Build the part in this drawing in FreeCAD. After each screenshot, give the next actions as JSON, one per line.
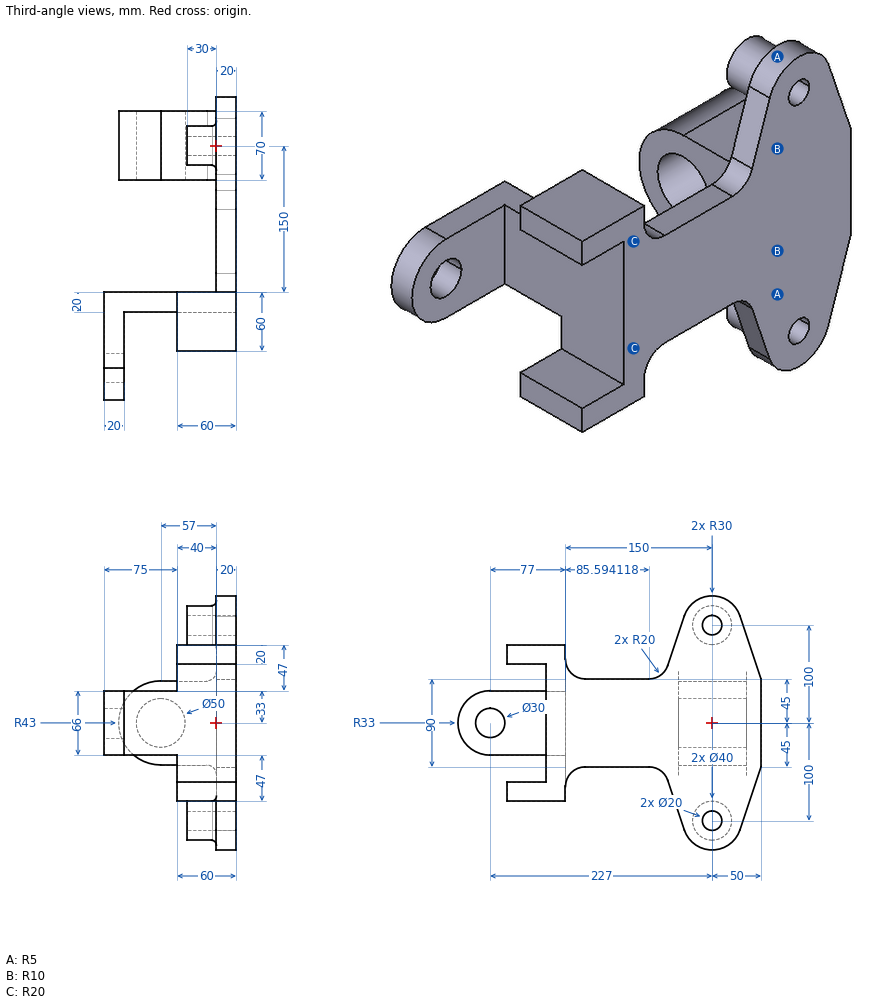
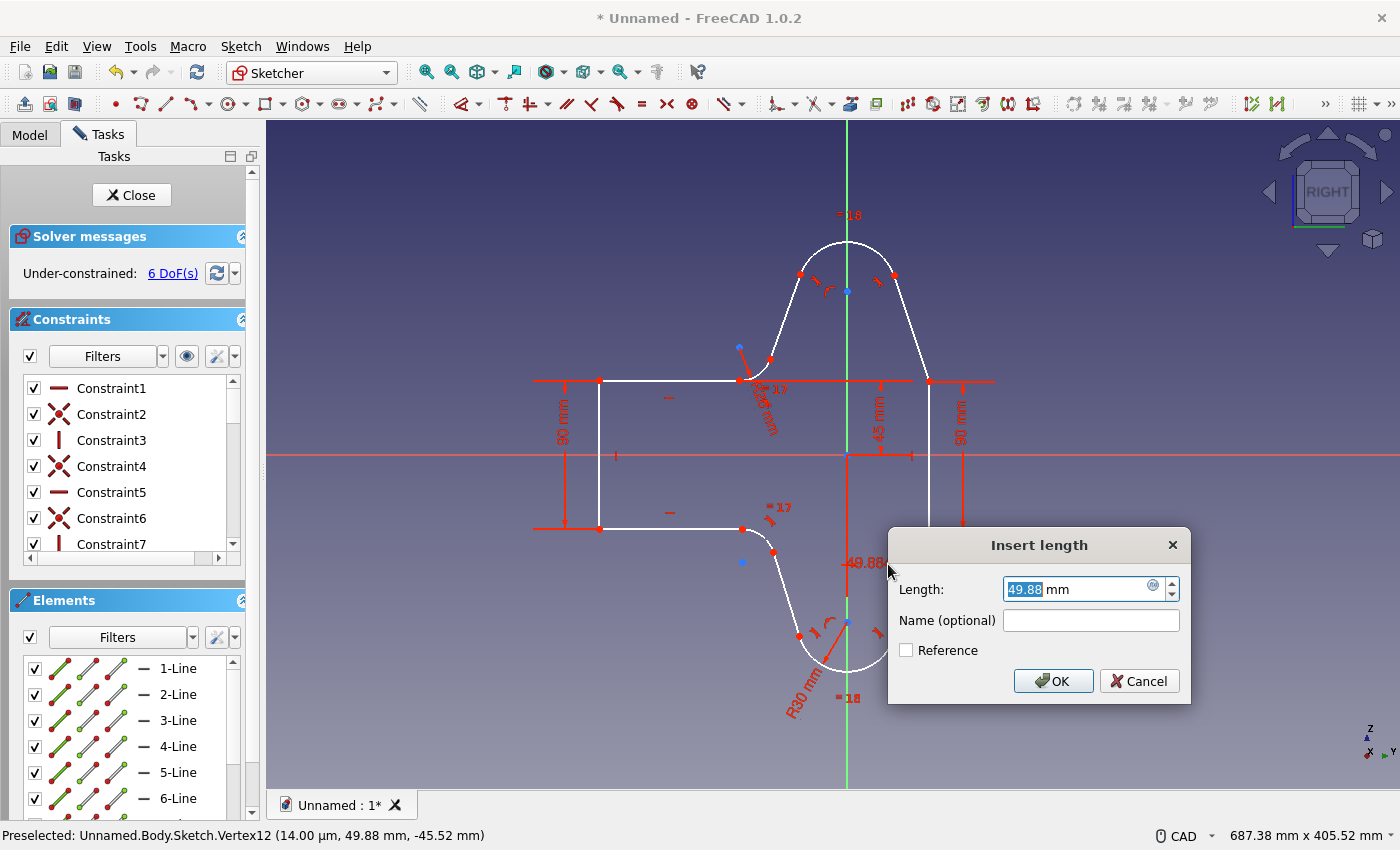
{"action": "type", "text": "50"}
{"action": "key", "text": "Return"}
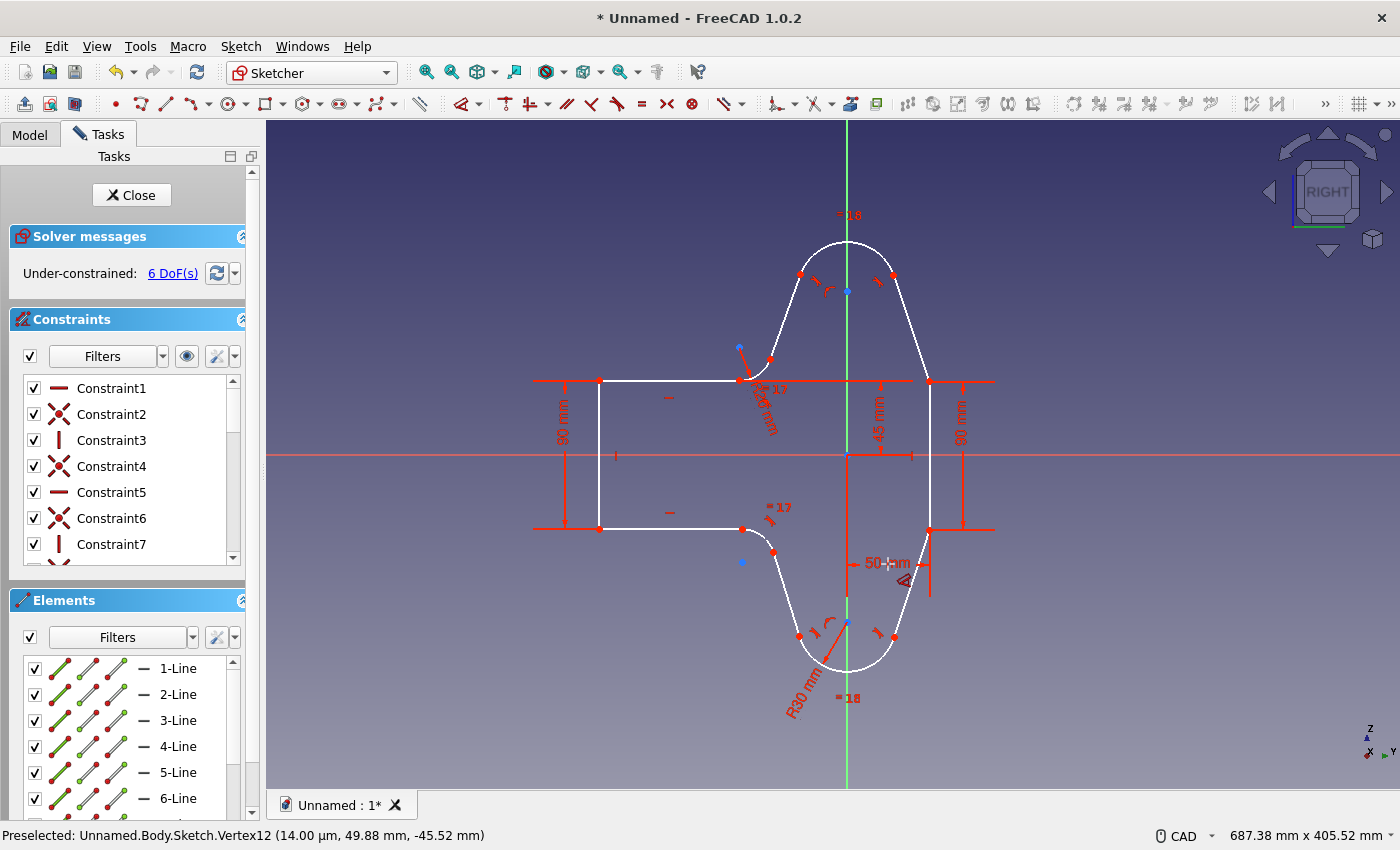
{"action": "left_click", "coordinate": [930, 530]}
{"action": "left_click", "coordinate": [964, 493]}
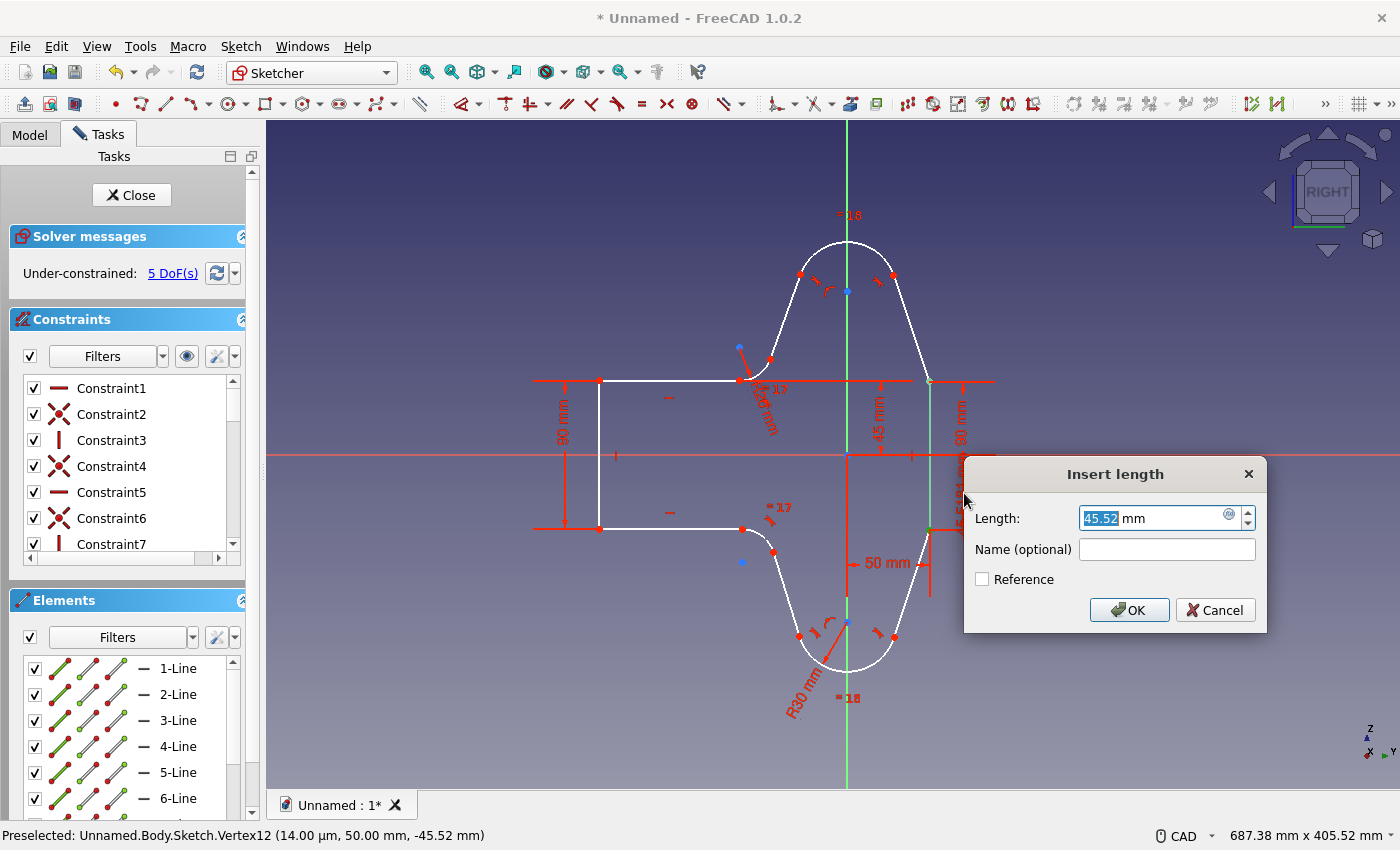
{"action": "type", "text": "45"}
{"action": "key", "text": "Return"}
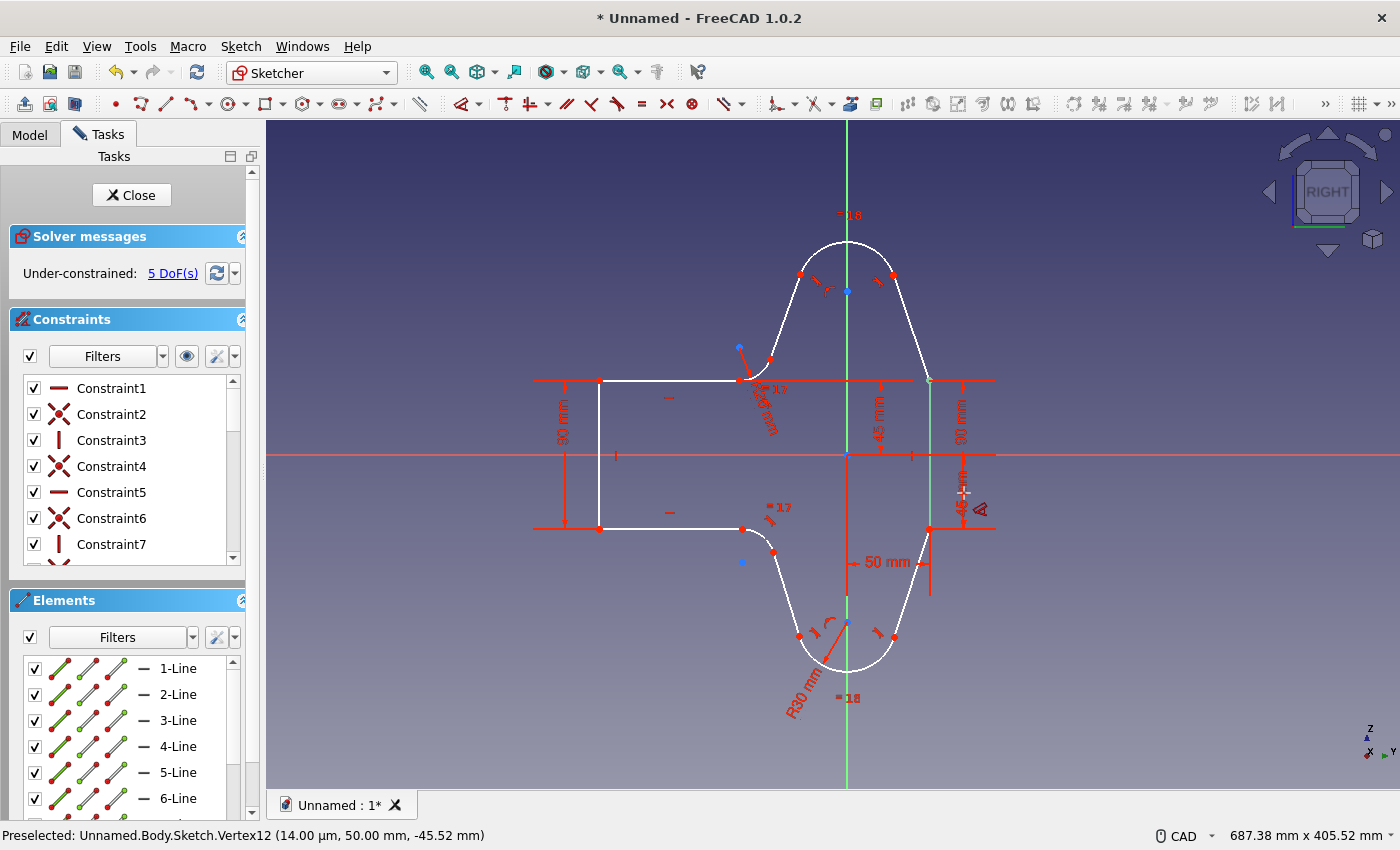
{"action": "left_click", "coordinate": [599, 381]}
{"action": "left_click", "coordinate": [723, 347]}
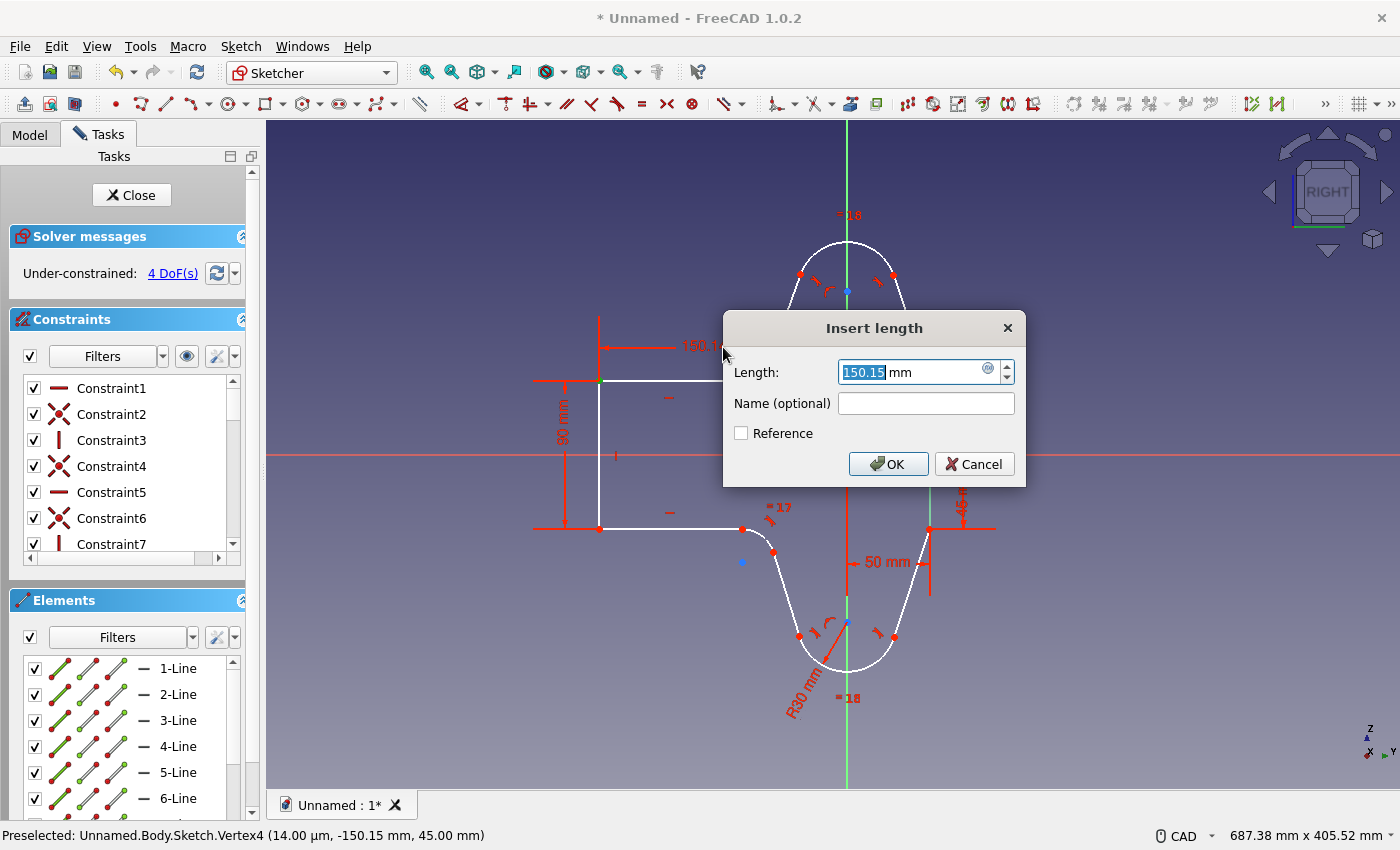
{"action": "type", "text": "150"}
{"action": "key", "text": "Return"}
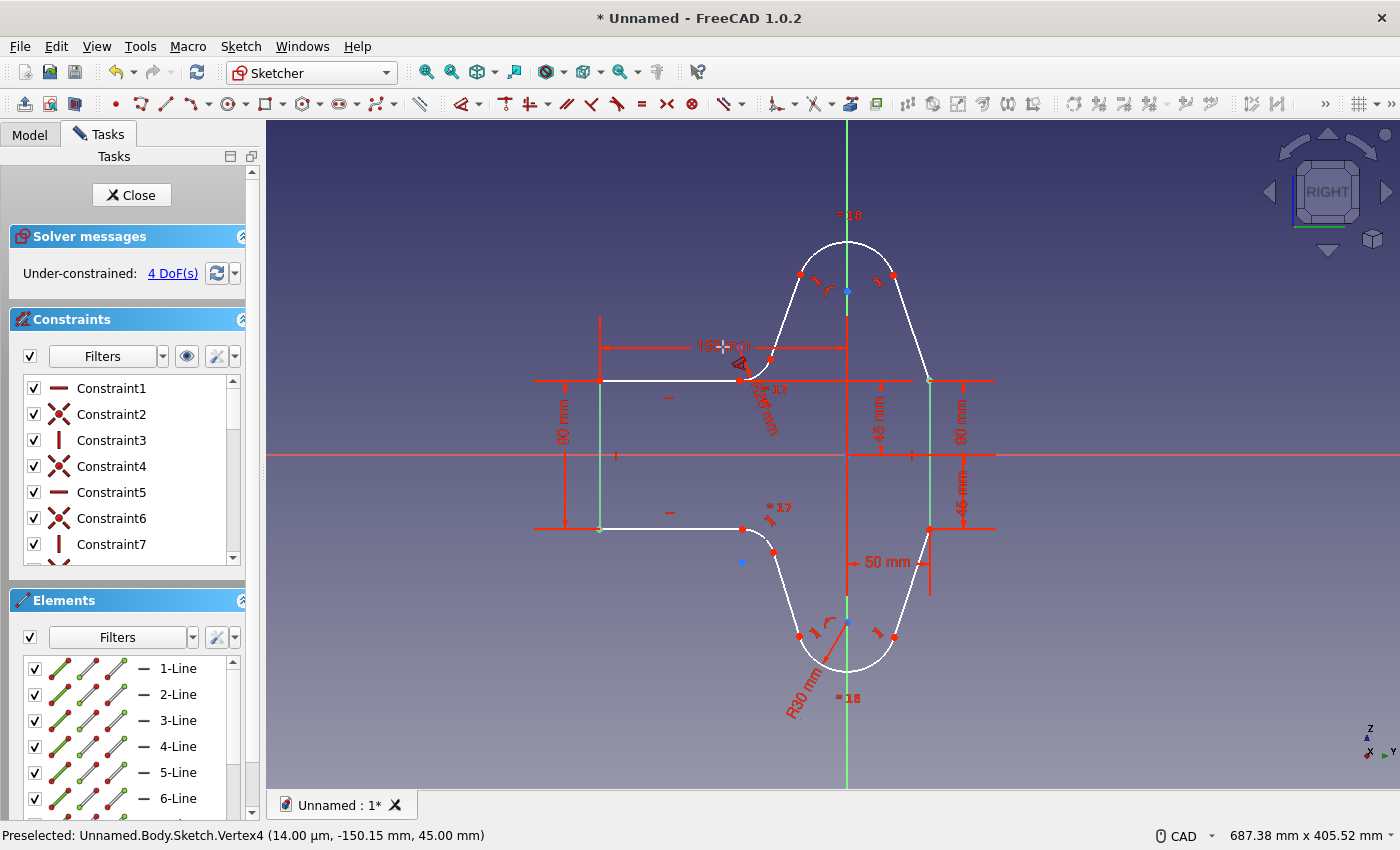
{"action": "left_click", "coordinate": [847, 622]}
{"action": "left_click", "coordinate": [881, 539]}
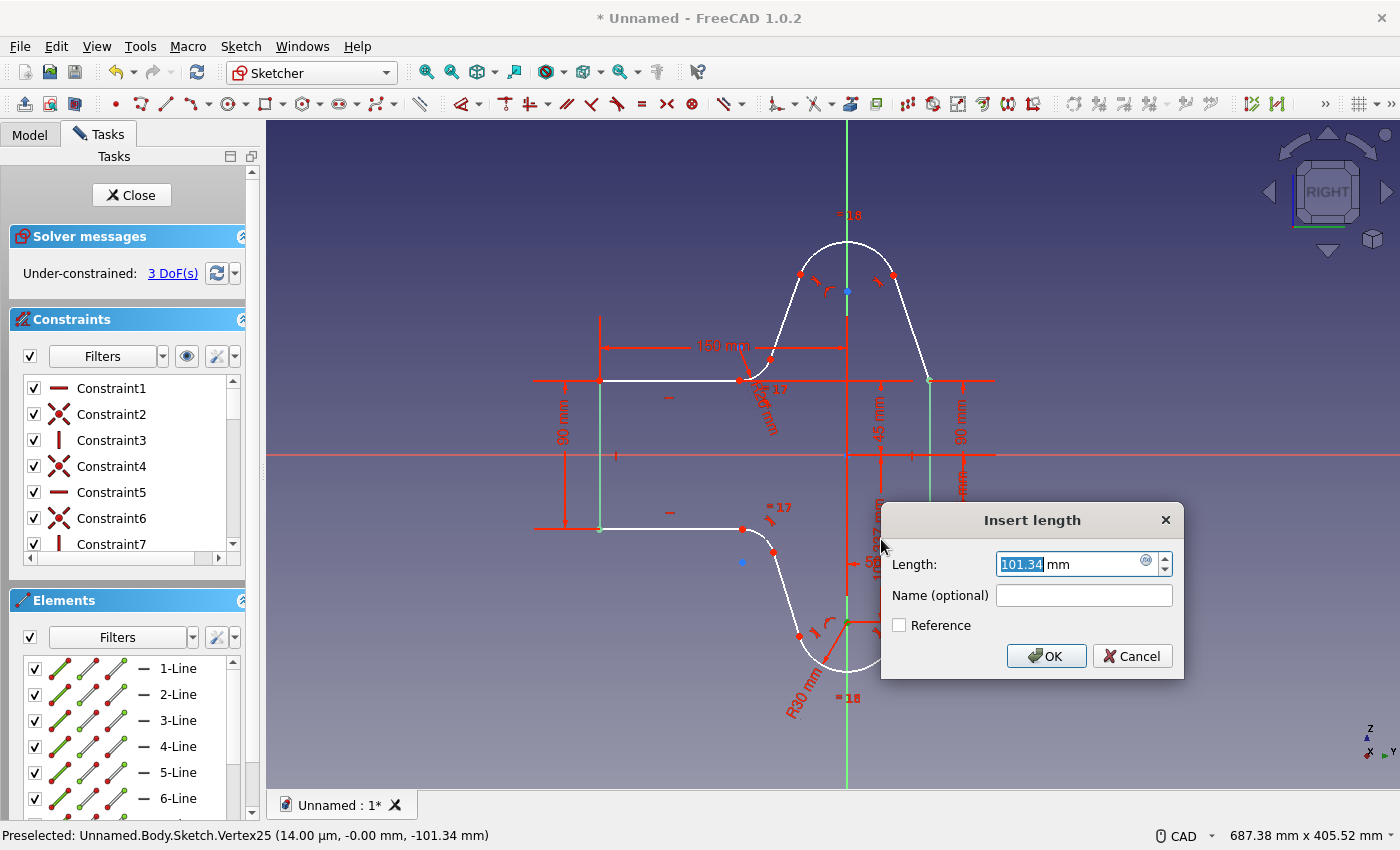
{"action": "type", "text": "100"}
{"action": "key", "text": "Return"}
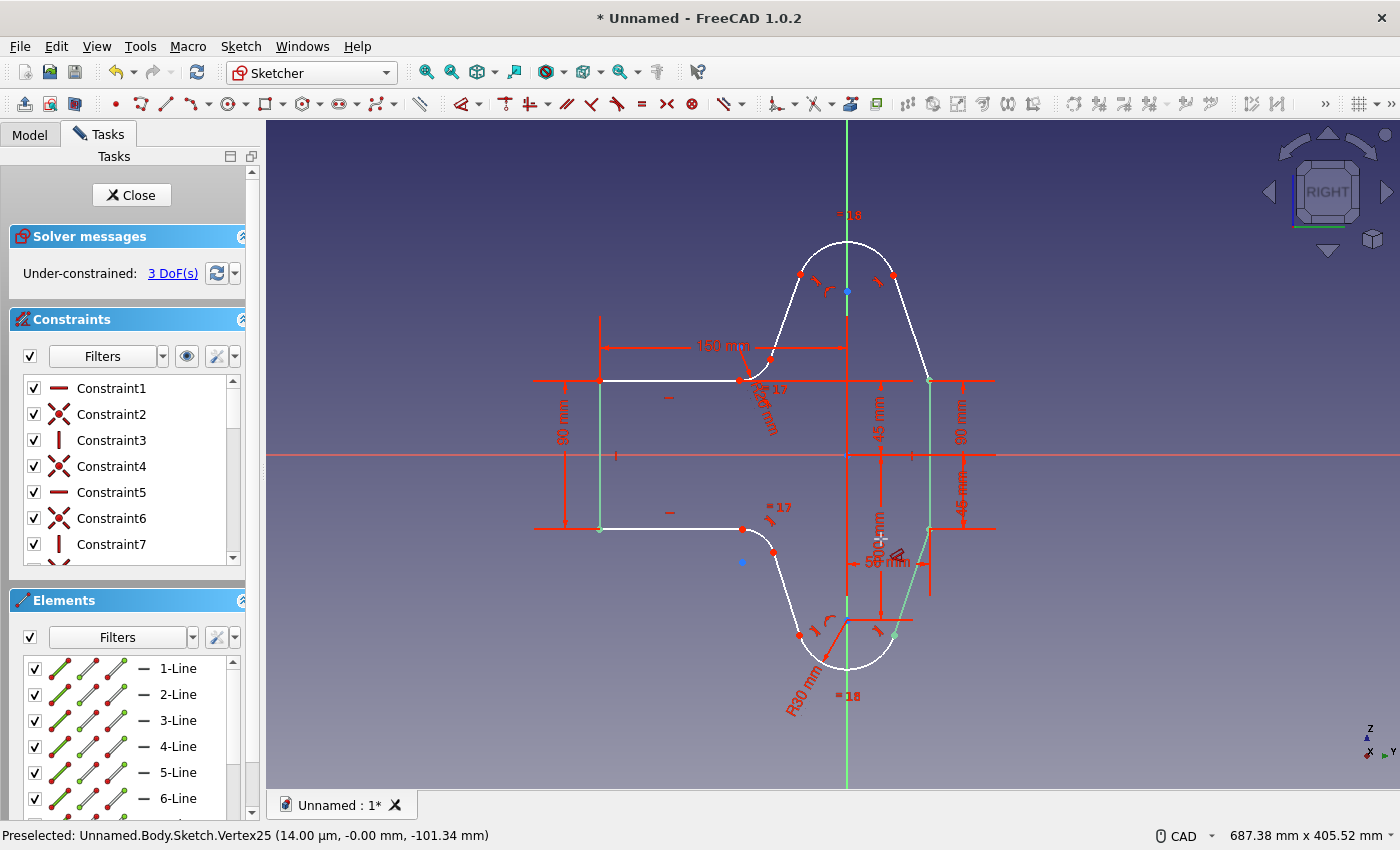
{"action": "left_click", "coordinate": [847, 292]}
{"action": "left_click", "coordinate": [881, 373]}